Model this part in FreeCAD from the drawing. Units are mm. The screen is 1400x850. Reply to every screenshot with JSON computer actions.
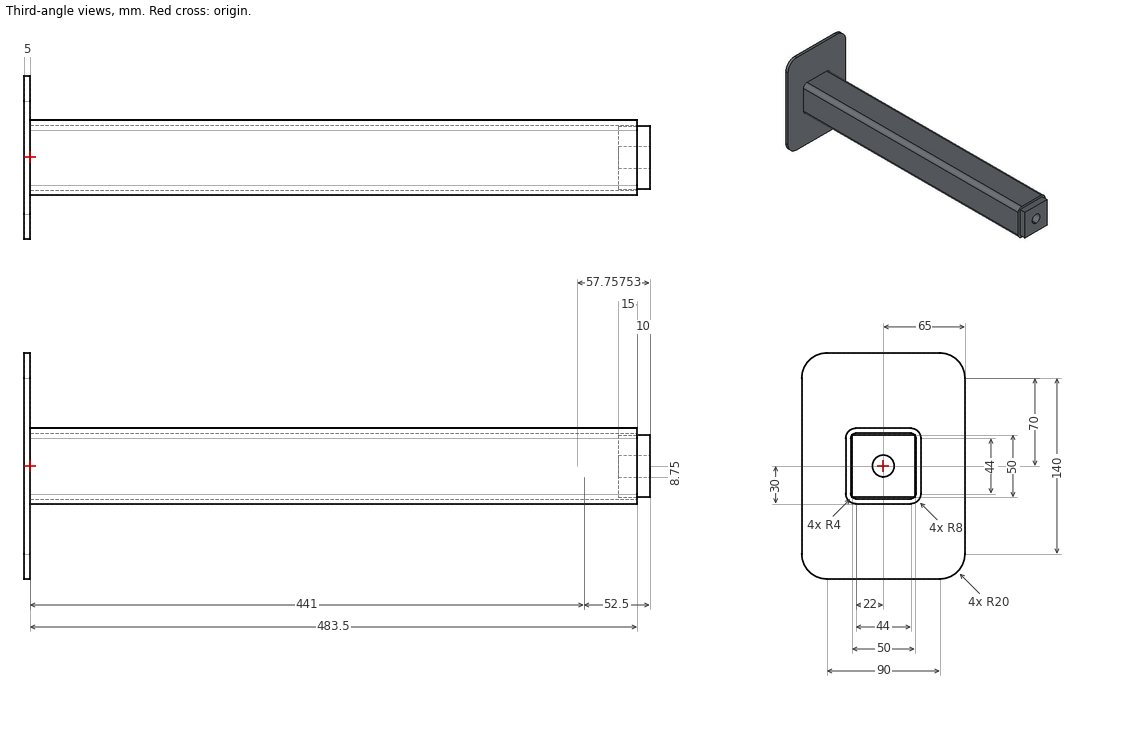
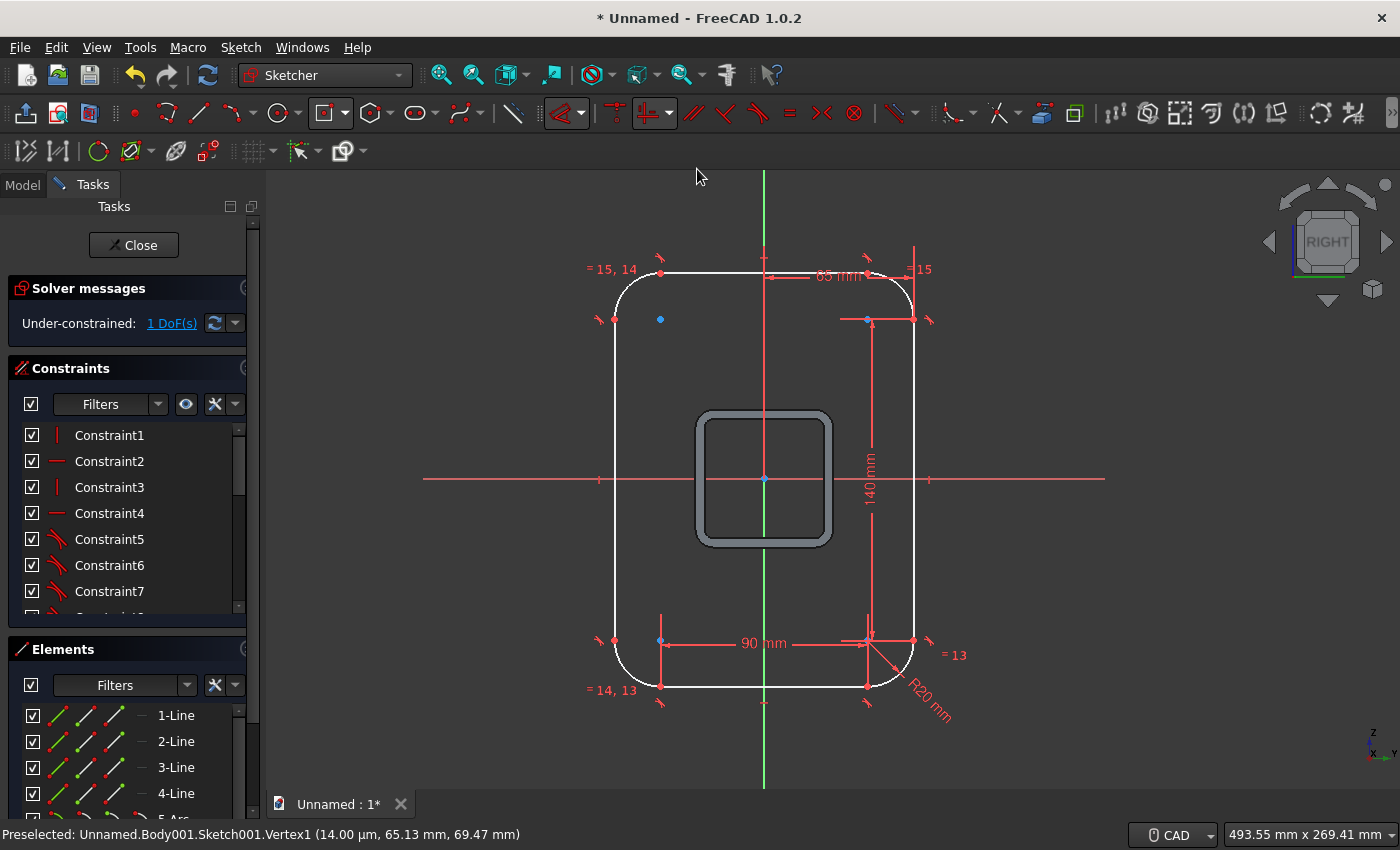
{"action": "left_click", "coordinate": [914, 319]}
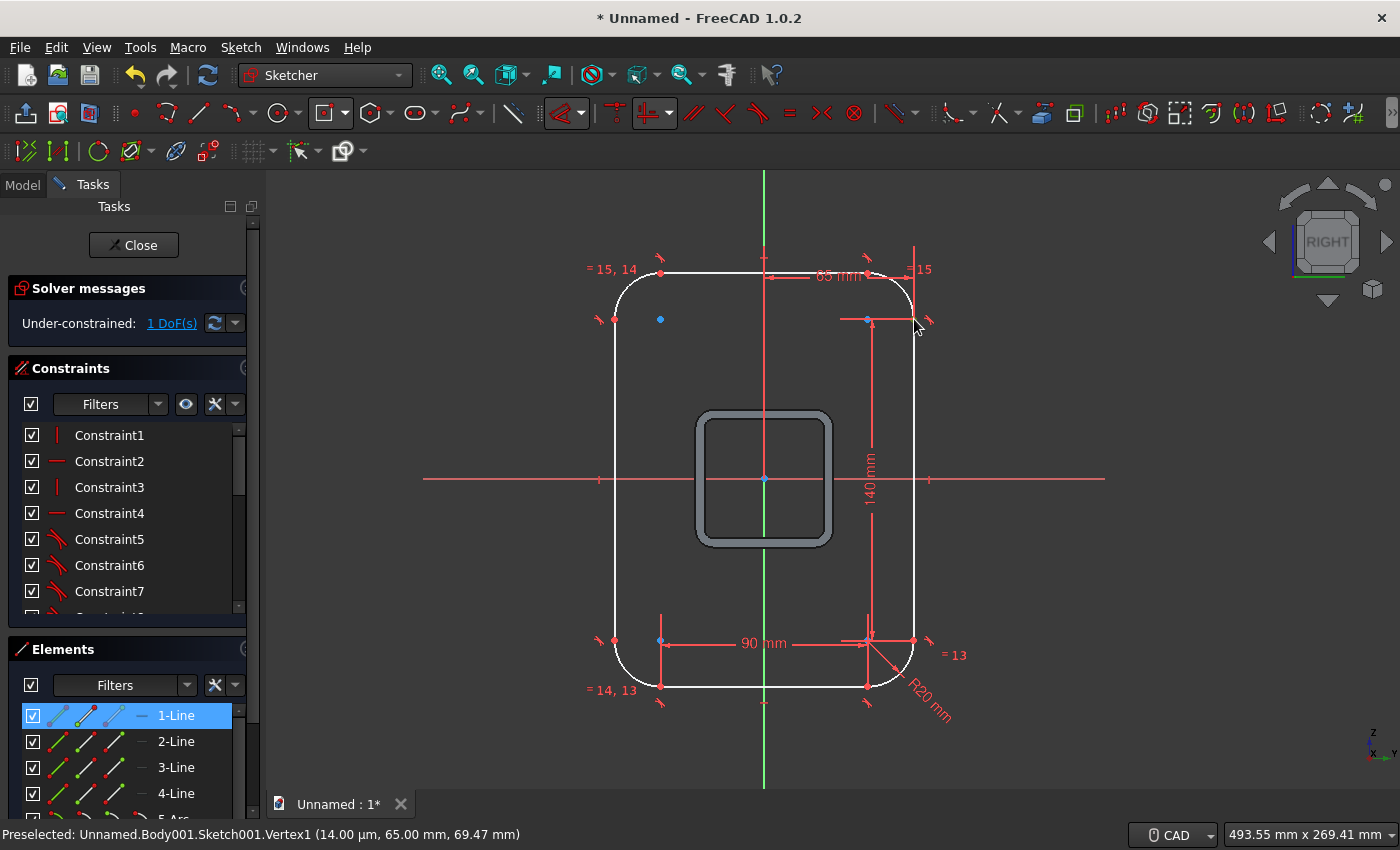
{"action": "key", "text": "i"}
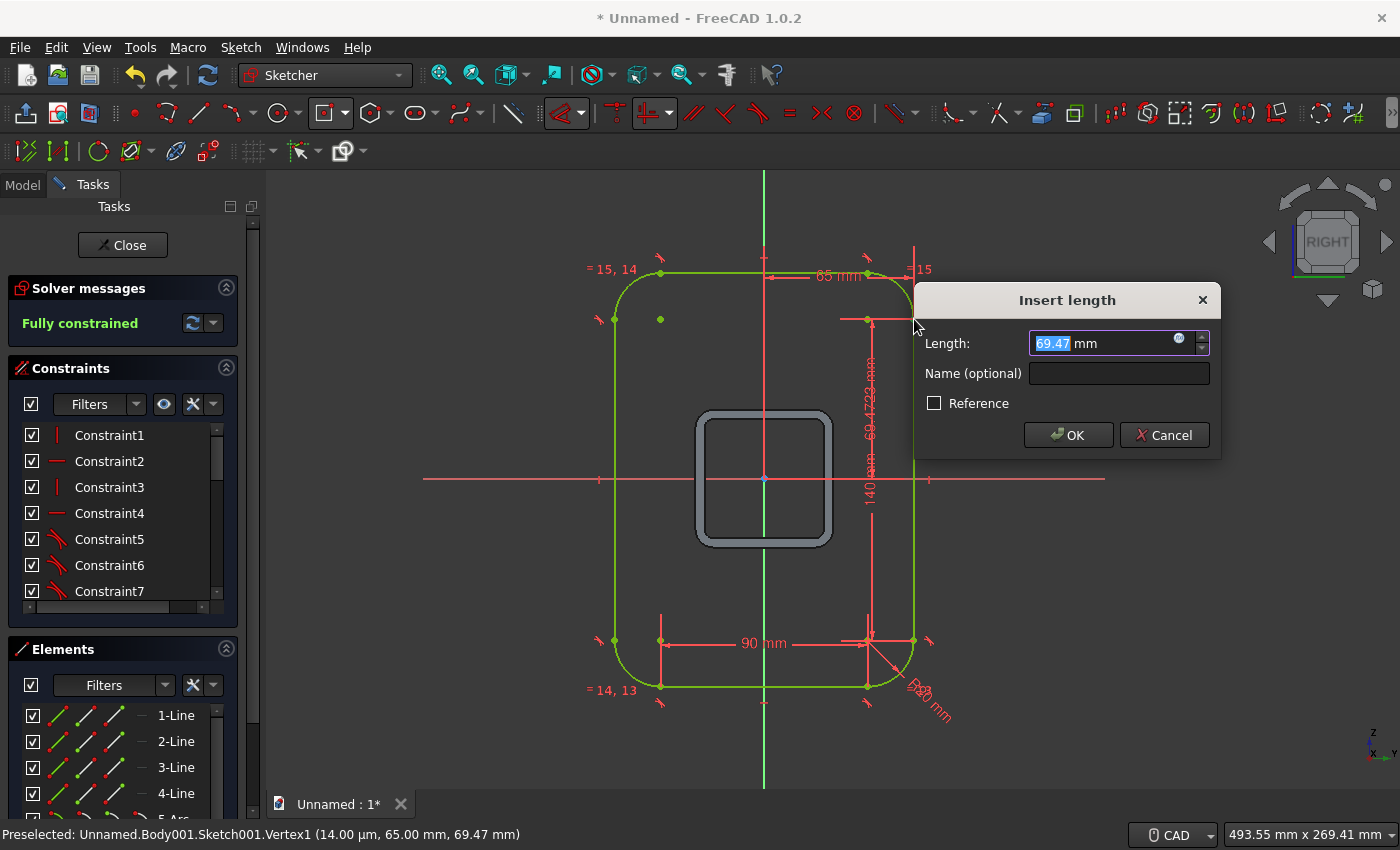
{"action": "type", "text": "70"}
{"action": "key", "text": "Return"}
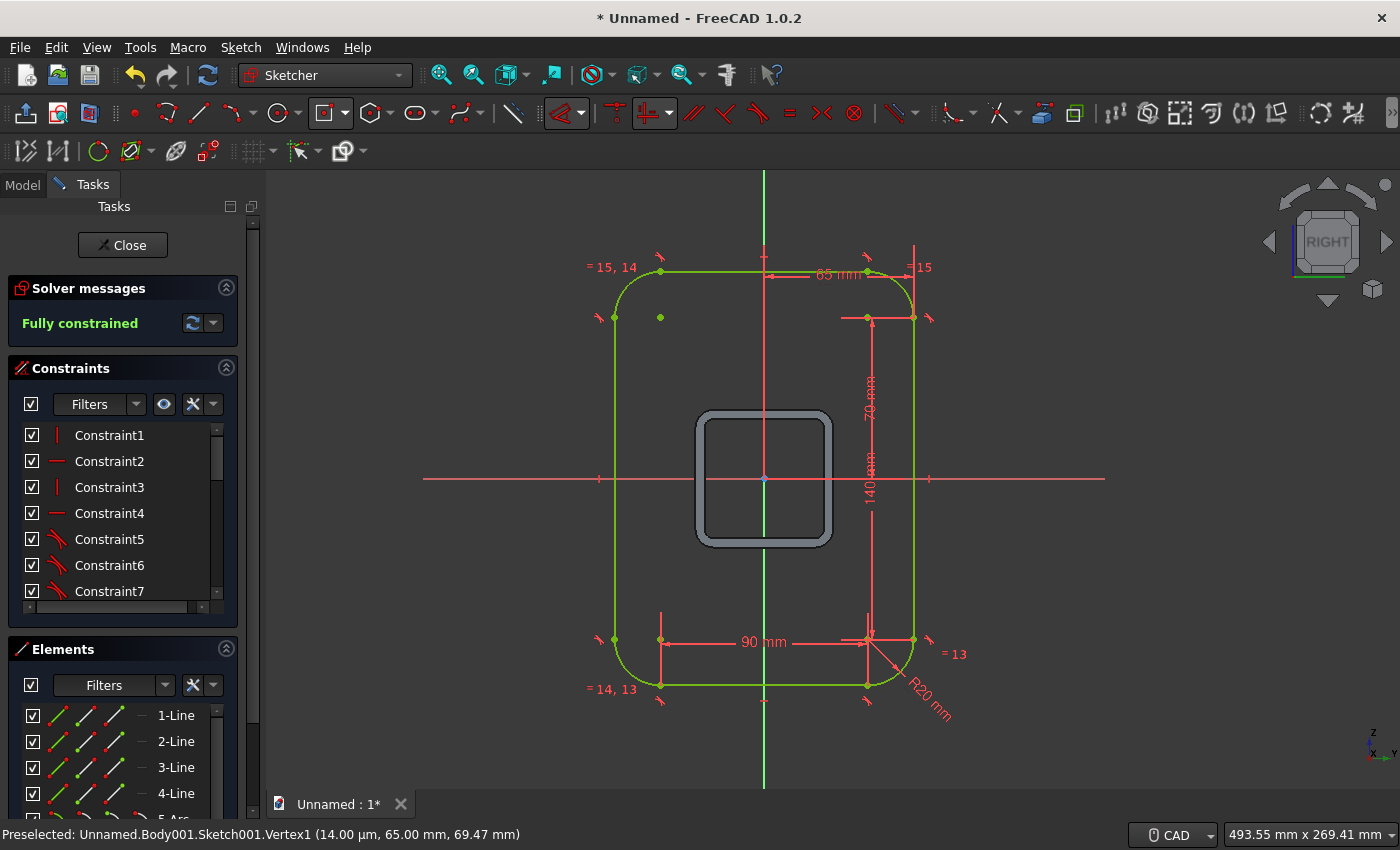
{"action": "left_click", "coordinate": [123, 245]}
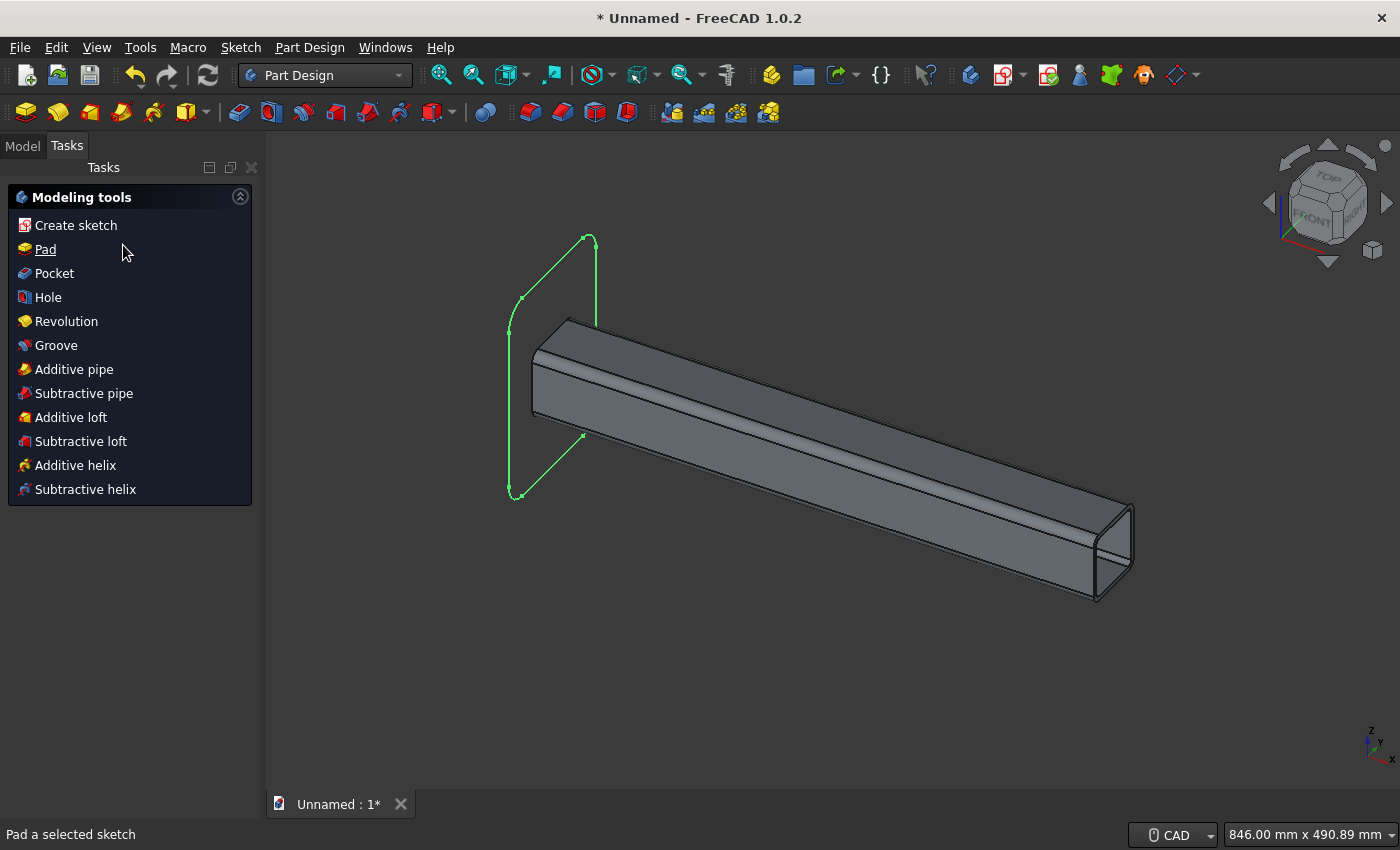
{"action": "left_click", "coordinate": [26, 112]}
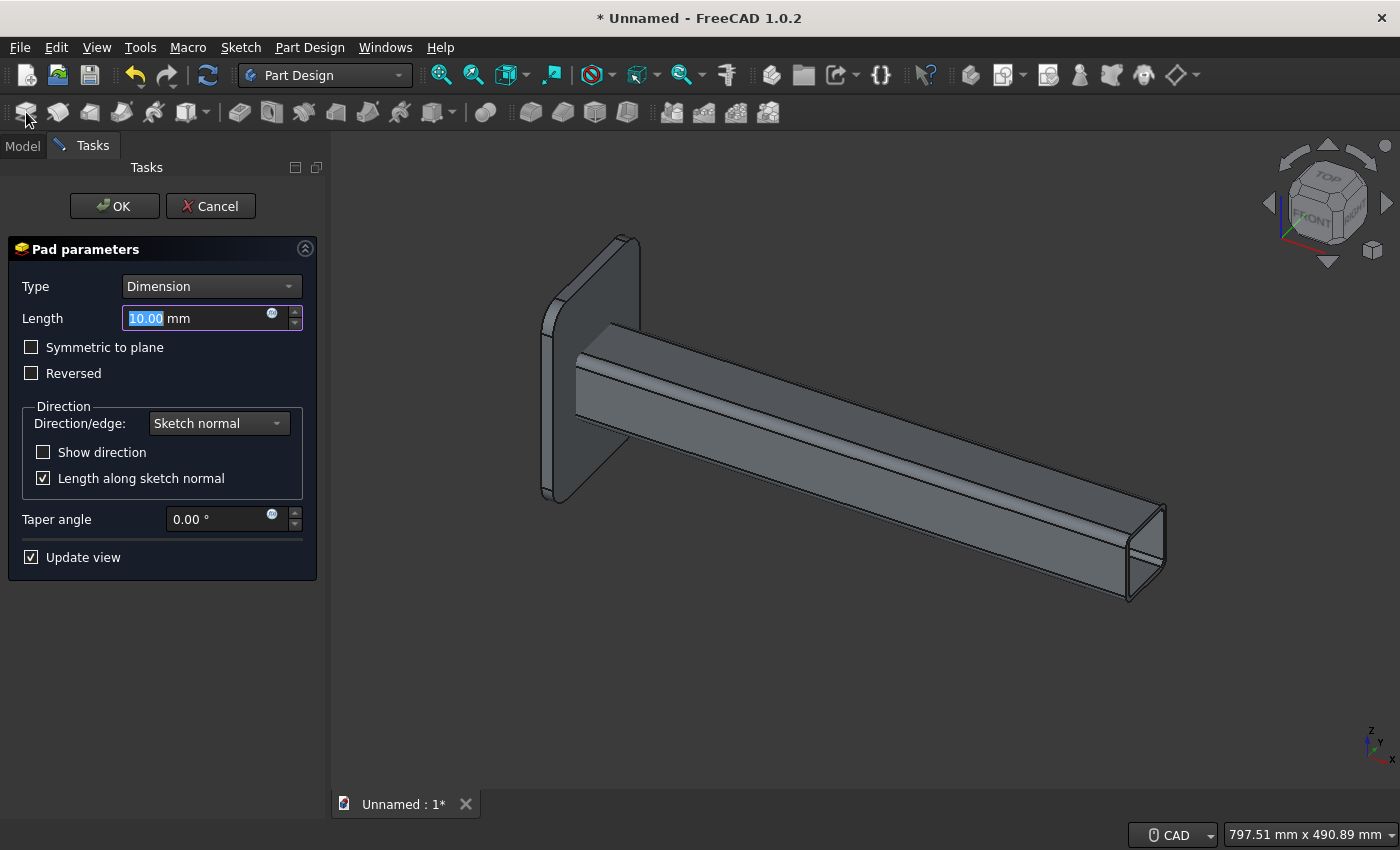
{"action": "type", "text": "5"}
{"action": "key", "text": "Tab"}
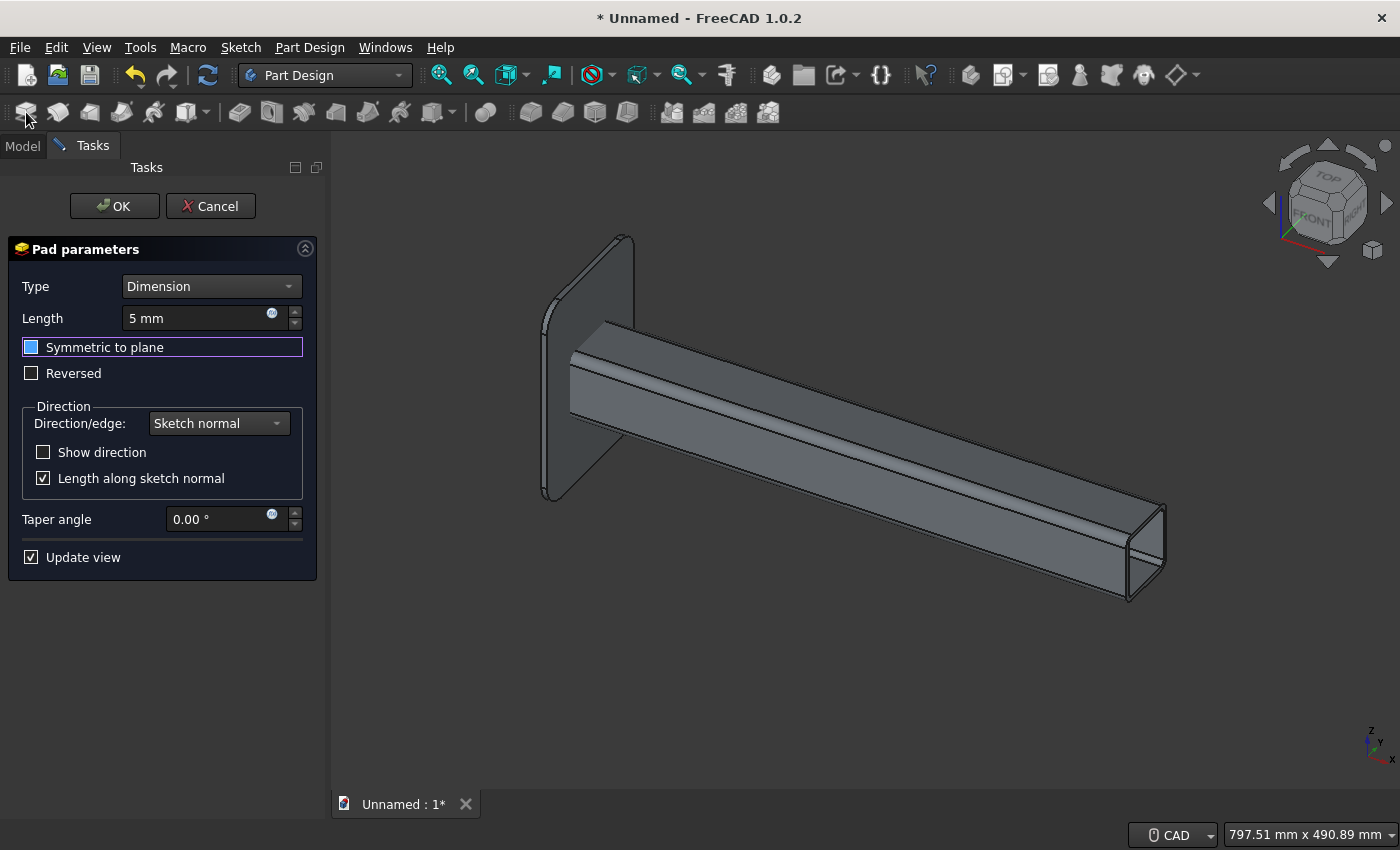
{"action": "left_click", "coordinate": [30, 373]}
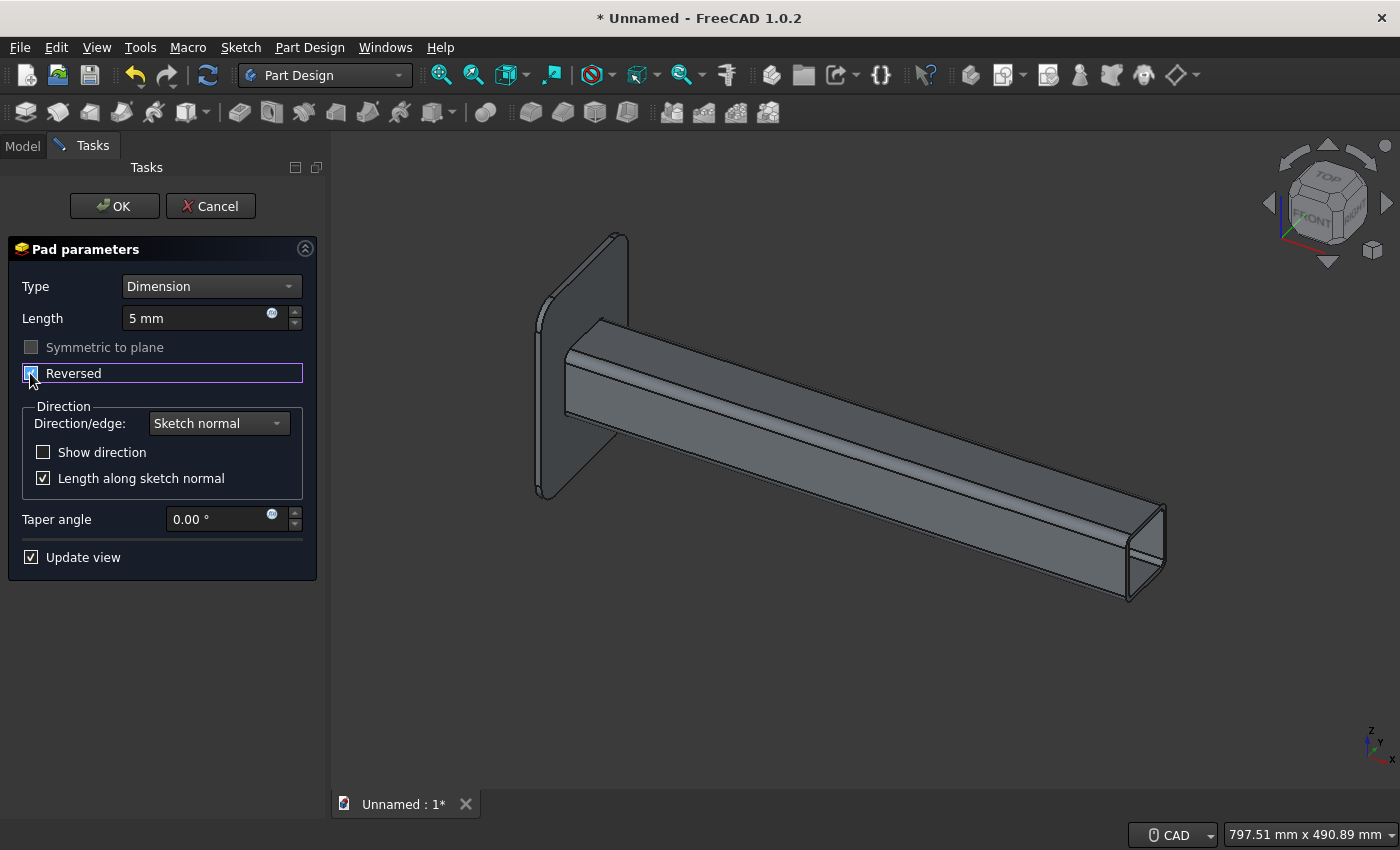
{"action": "left_click", "coordinate": [115, 206]}